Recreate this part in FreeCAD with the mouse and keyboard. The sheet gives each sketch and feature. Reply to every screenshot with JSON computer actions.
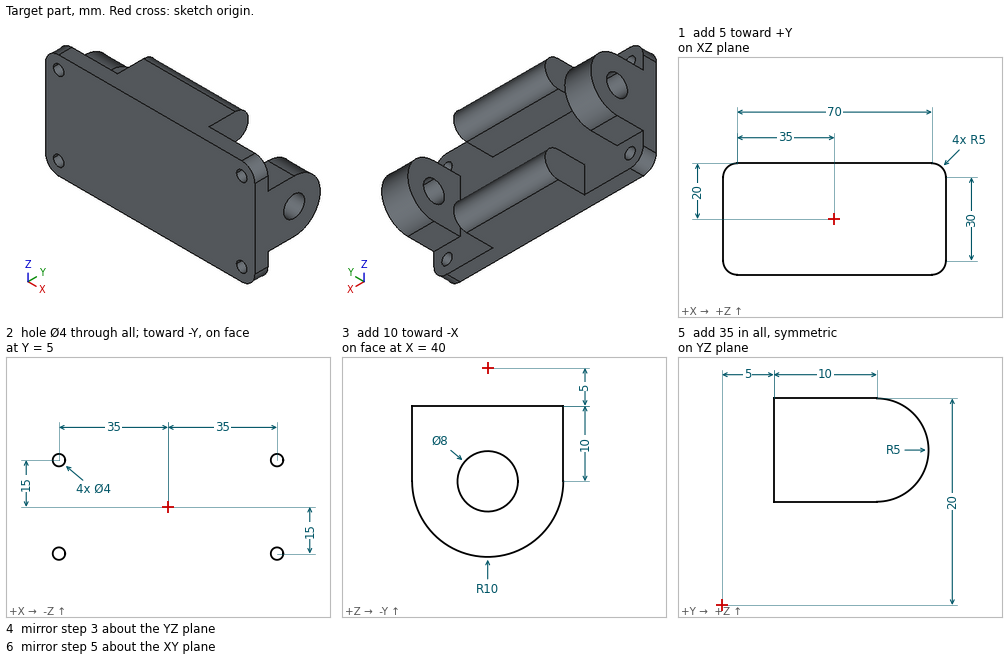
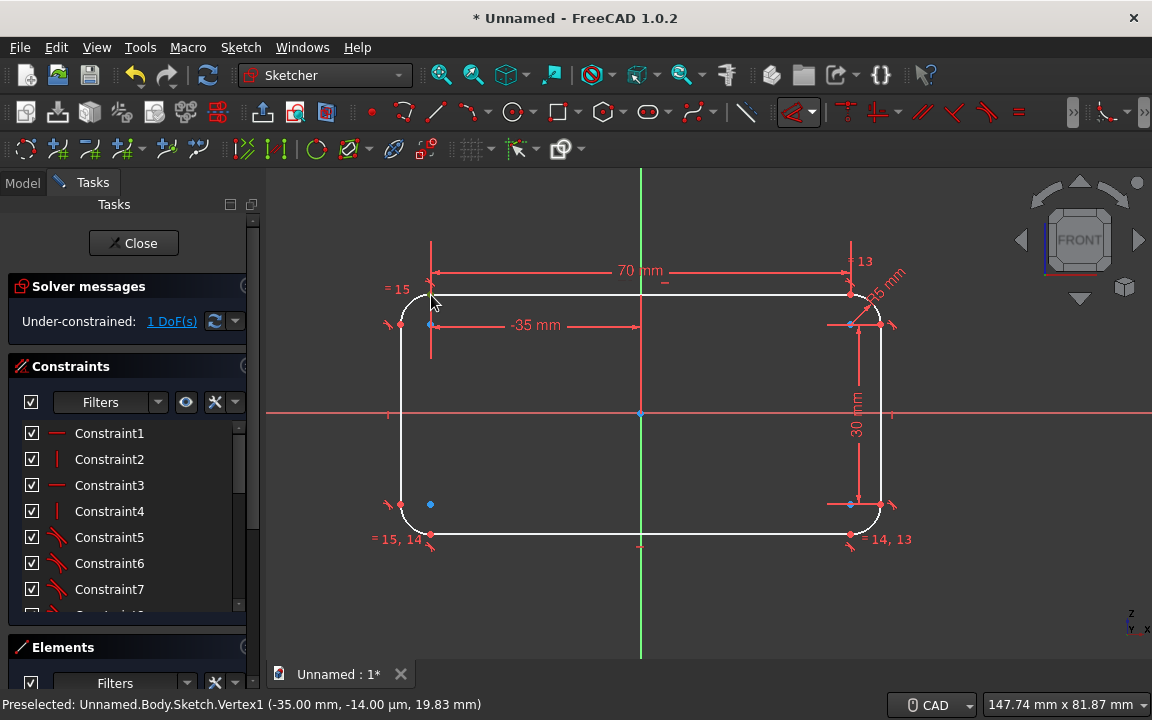
{"action": "key", "text": "i"}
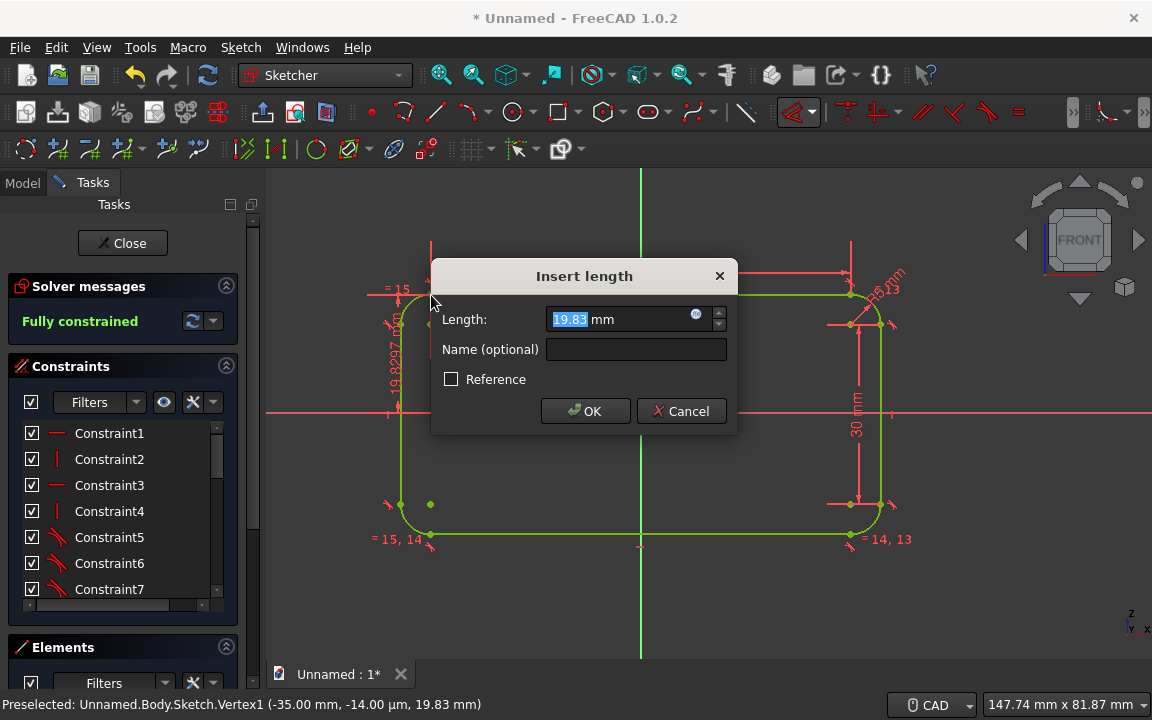
{"action": "type", "text": "20"}
{"action": "key", "text": "Return"}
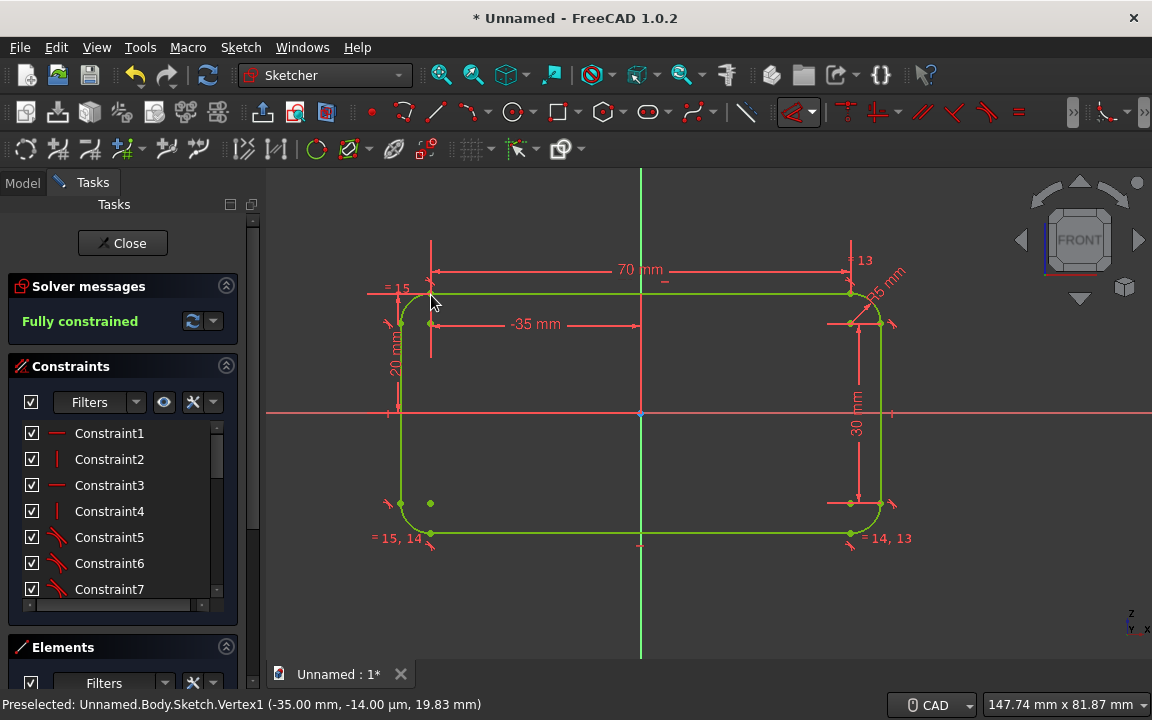
{"action": "left_click", "coordinate": [123, 243]}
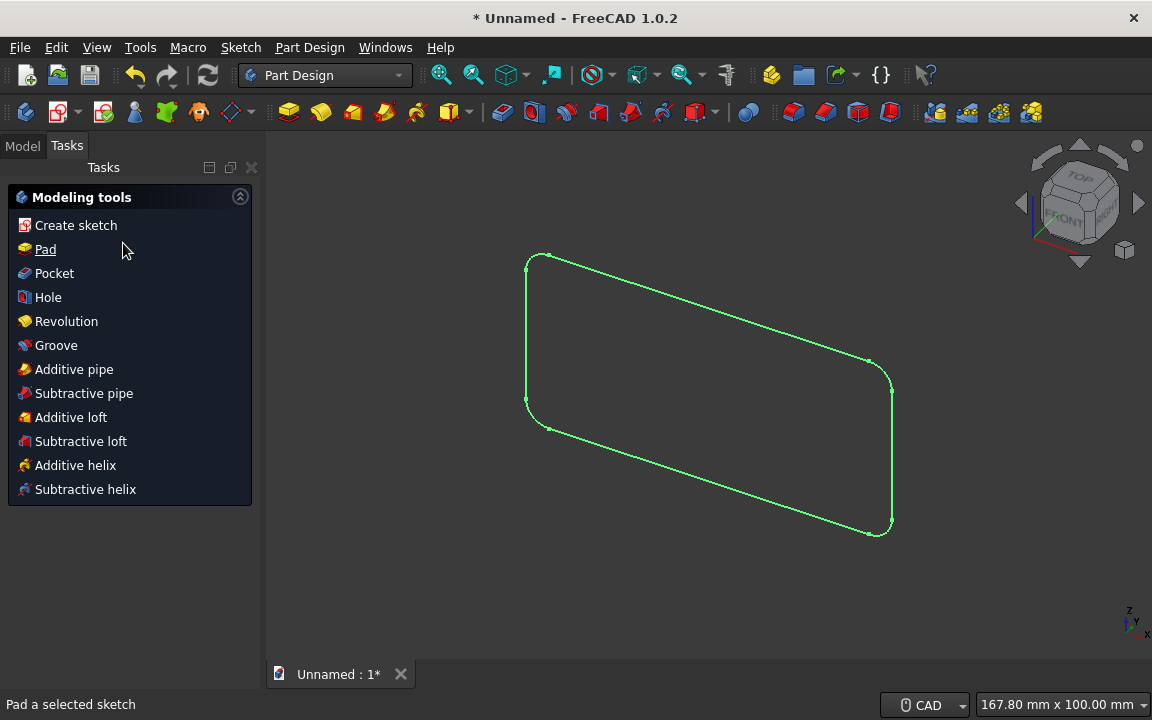
{"action": "left_click", "coordinate": [290, 112]}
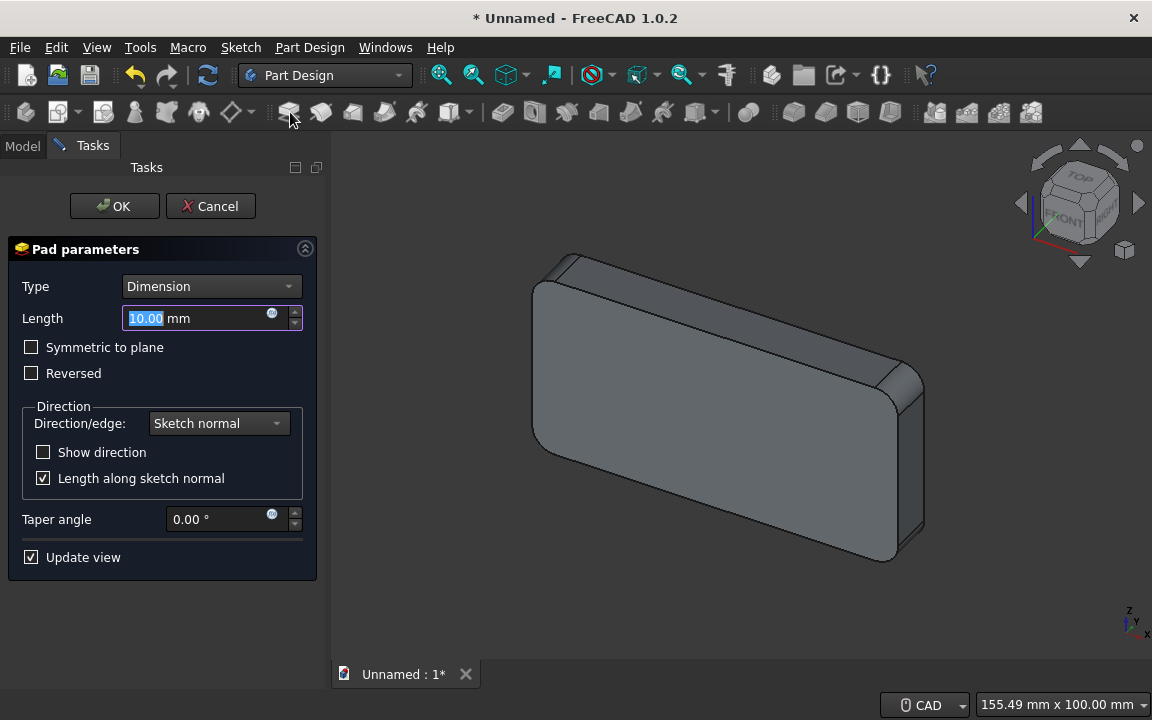
{"action": "type", "text": "5"}
{"action": "key", "text": "Tab"}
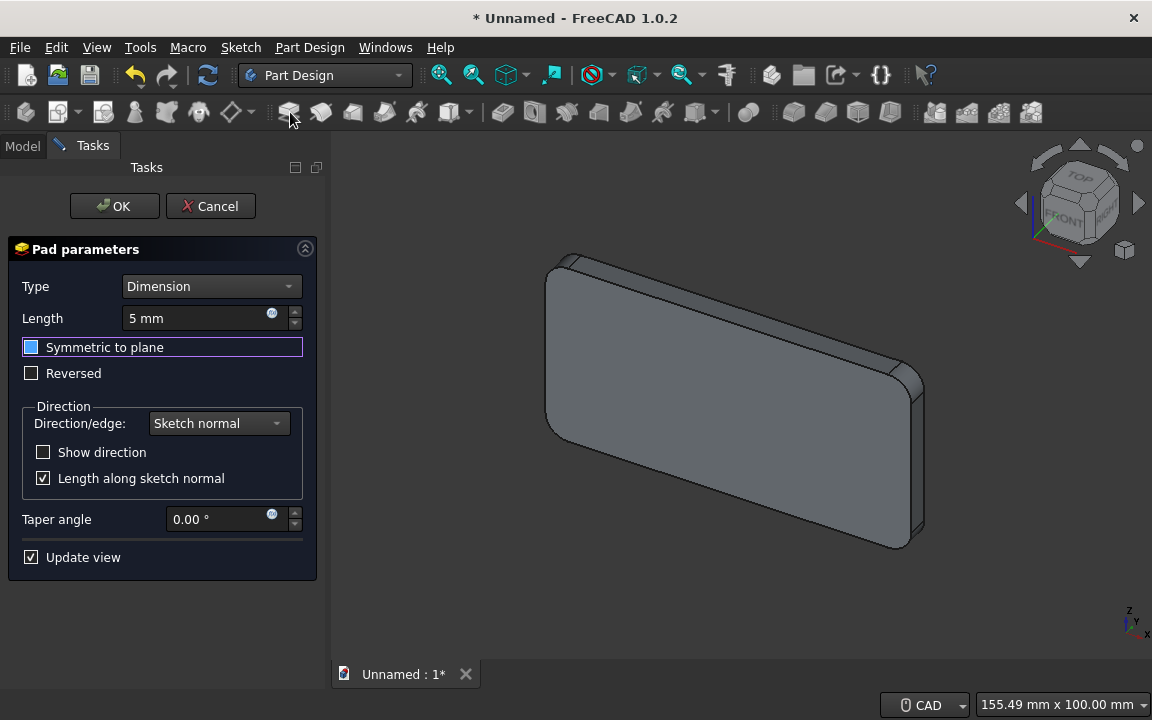
{"action": "left_click", "coordinate": [30, 373]}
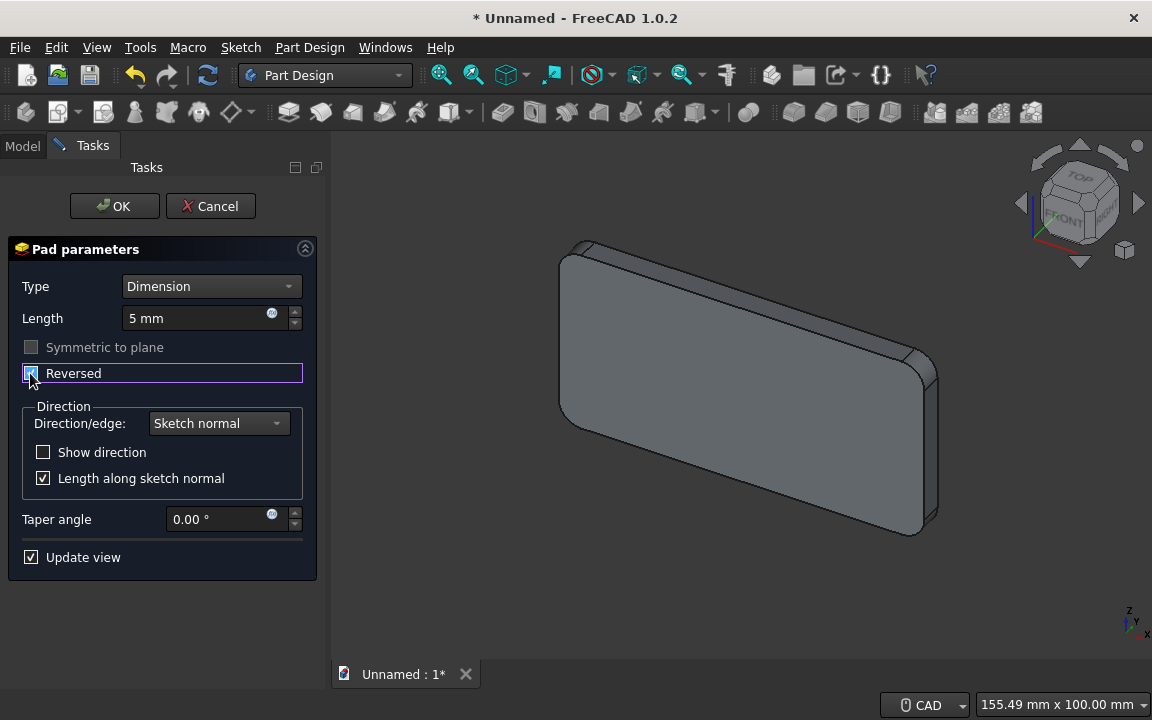
{"action": "left_click", "coordinate": [115, 206]}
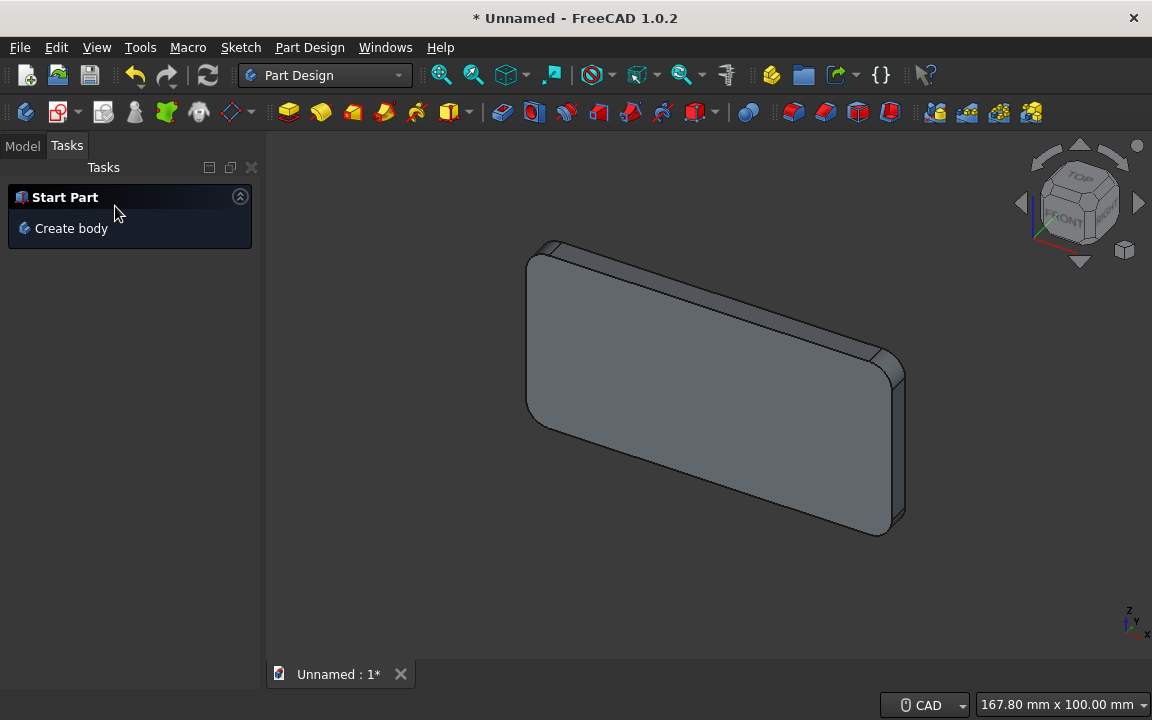
{"action": "key", "text": "4"}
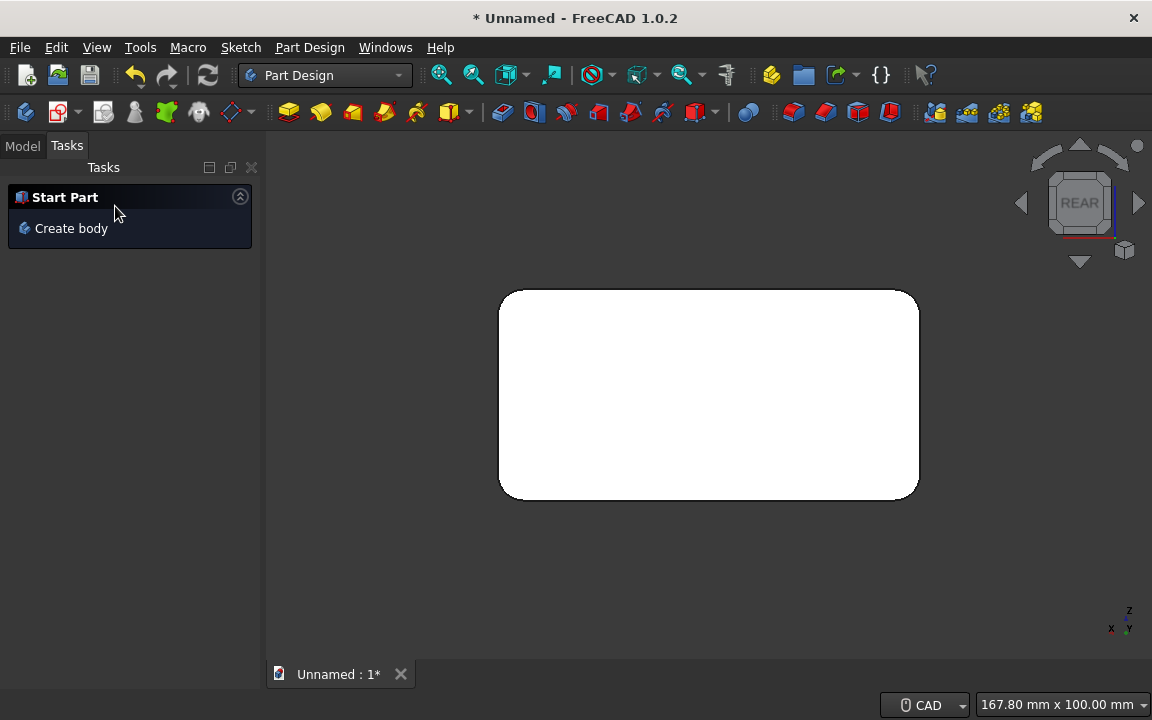
{"action": "left_click", "coordinate": [649, 394]}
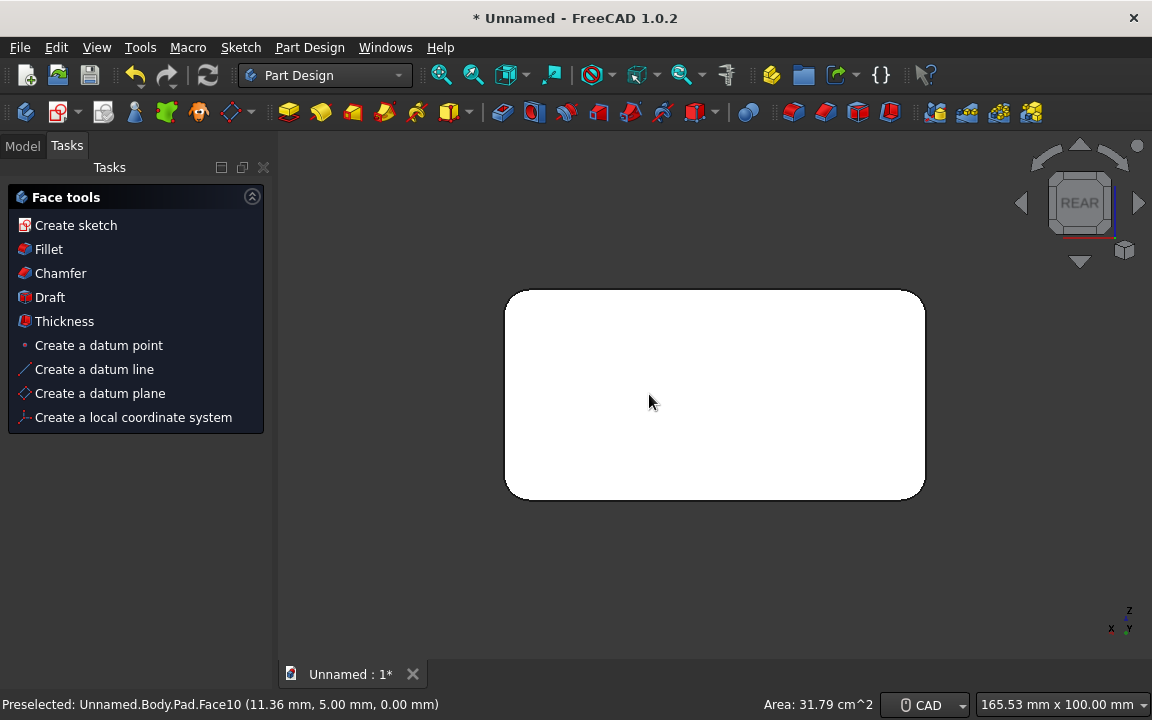
{"action": "left_click", "coordinate": [58, 112]}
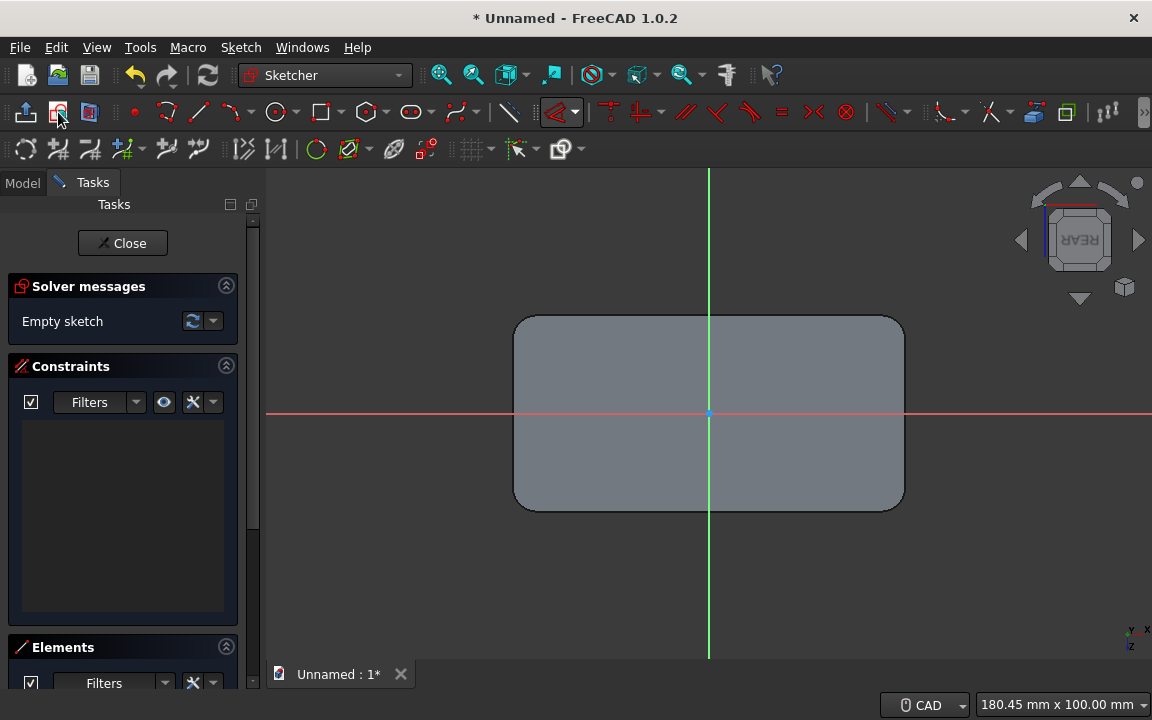
{"action": "left_click", "coordinate": [276, 112]}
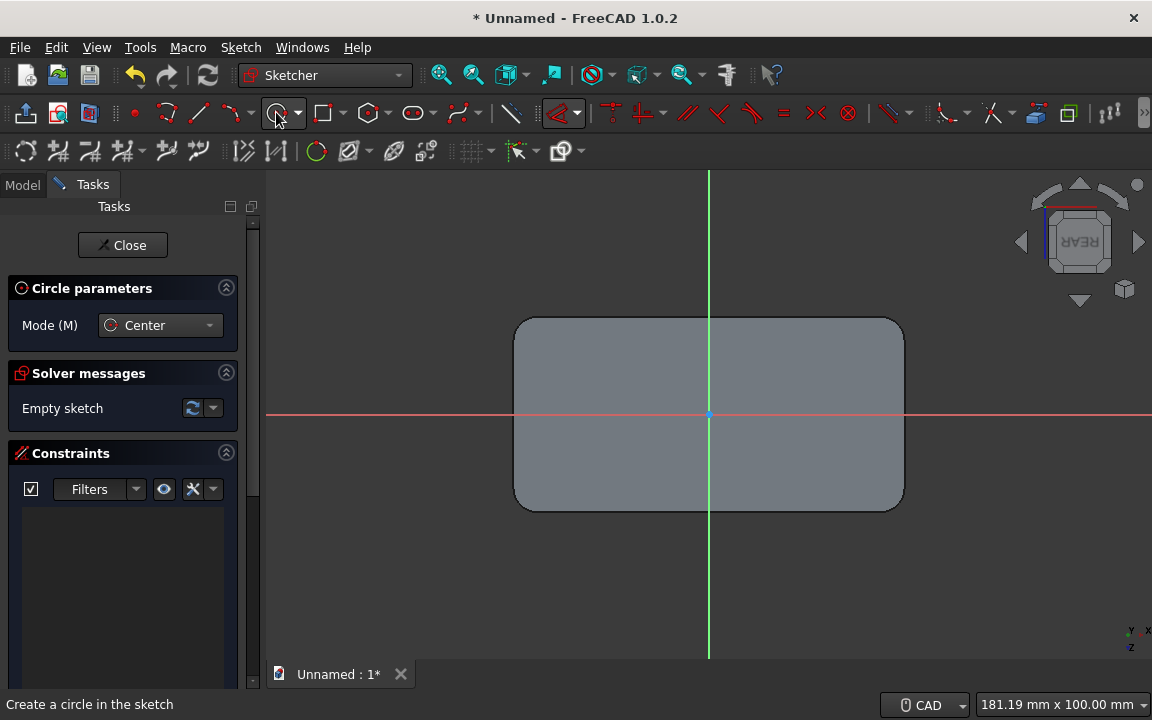
{"action": "scroll", "coordinate": [538, 341], "scroll_direction": "up", "scroll_amount": 5}